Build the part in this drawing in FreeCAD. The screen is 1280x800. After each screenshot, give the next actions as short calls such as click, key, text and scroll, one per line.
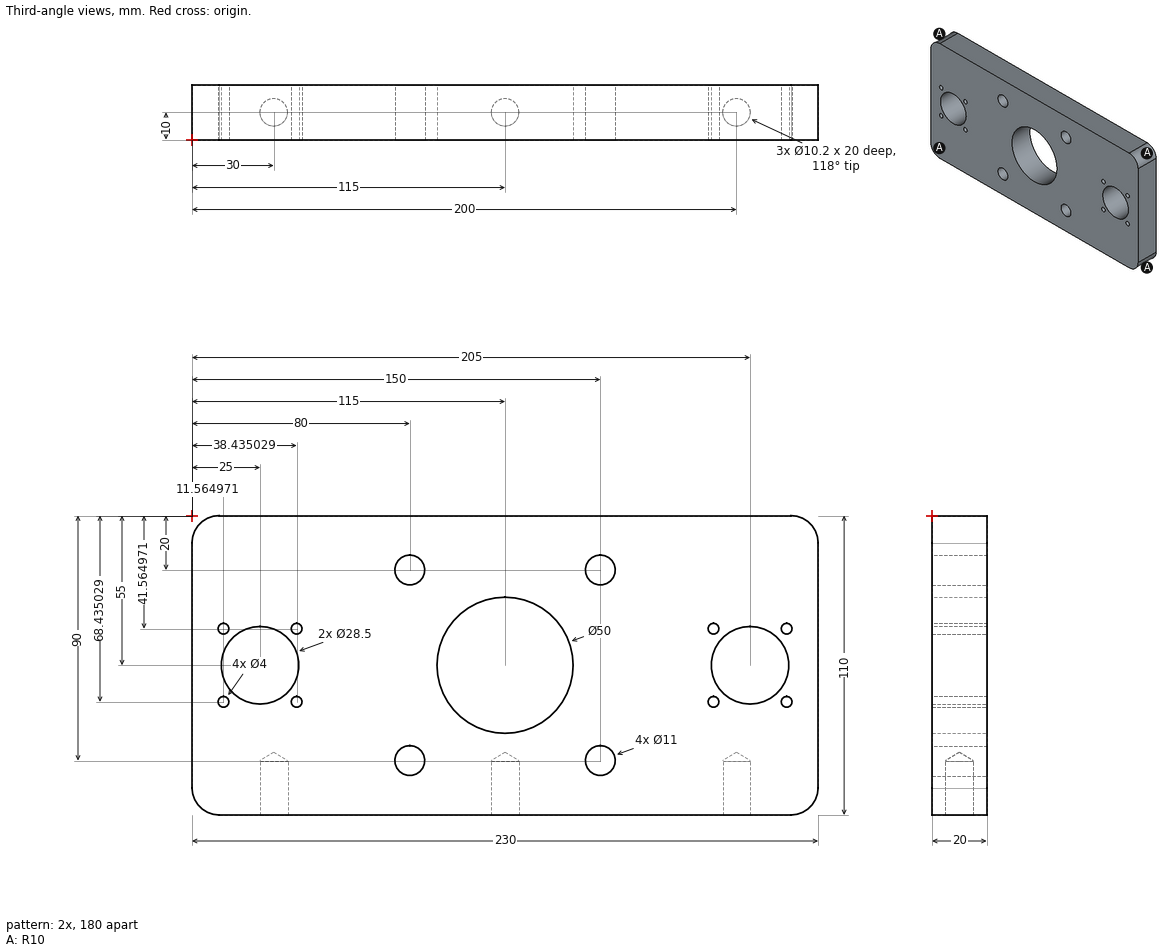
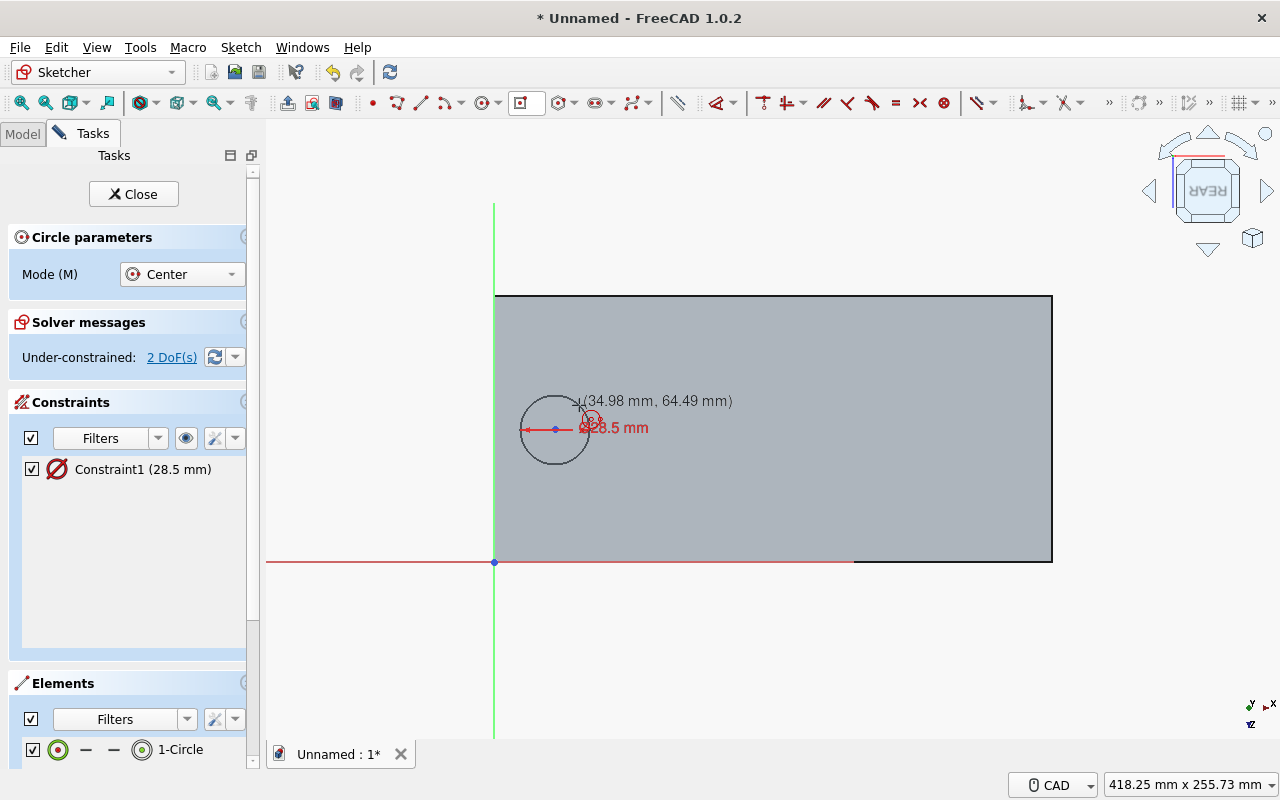
click(991, 429)
move(1016, 405)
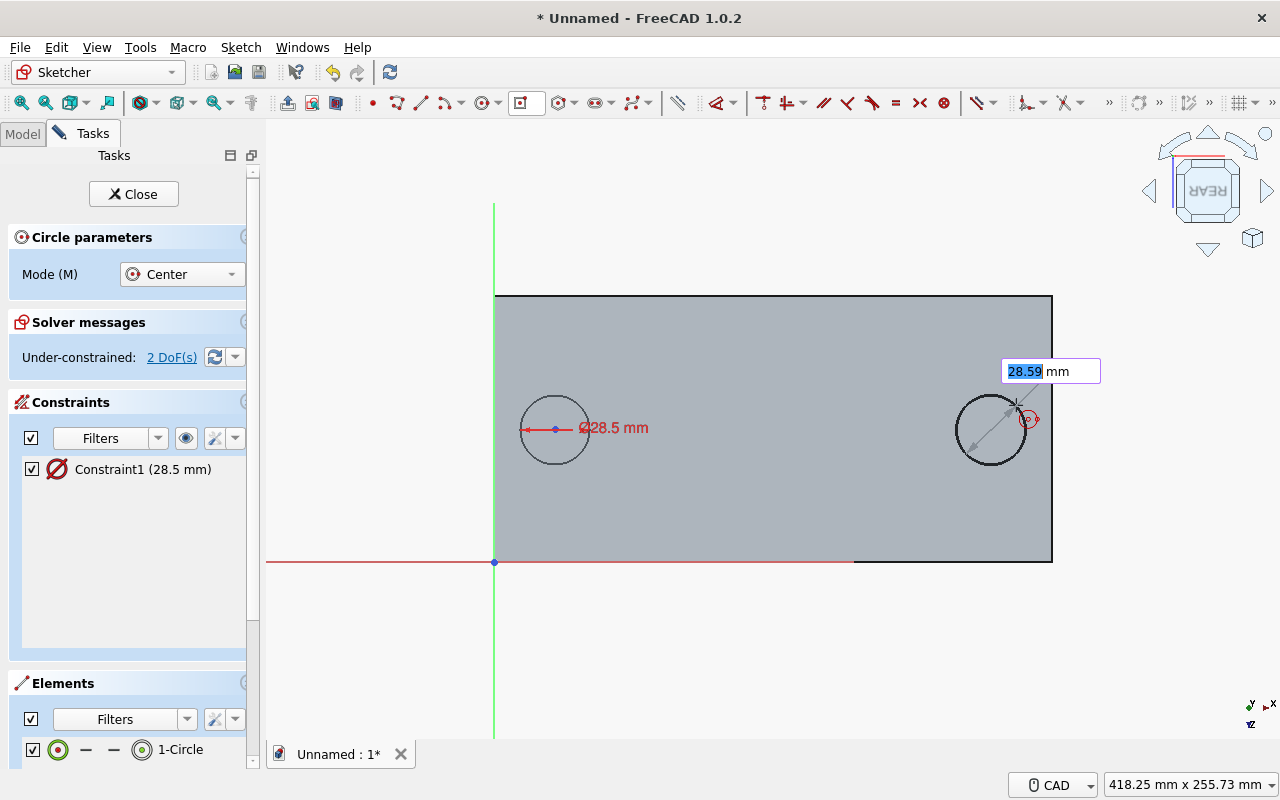
text(28.5)
key(Return)
key(Escape)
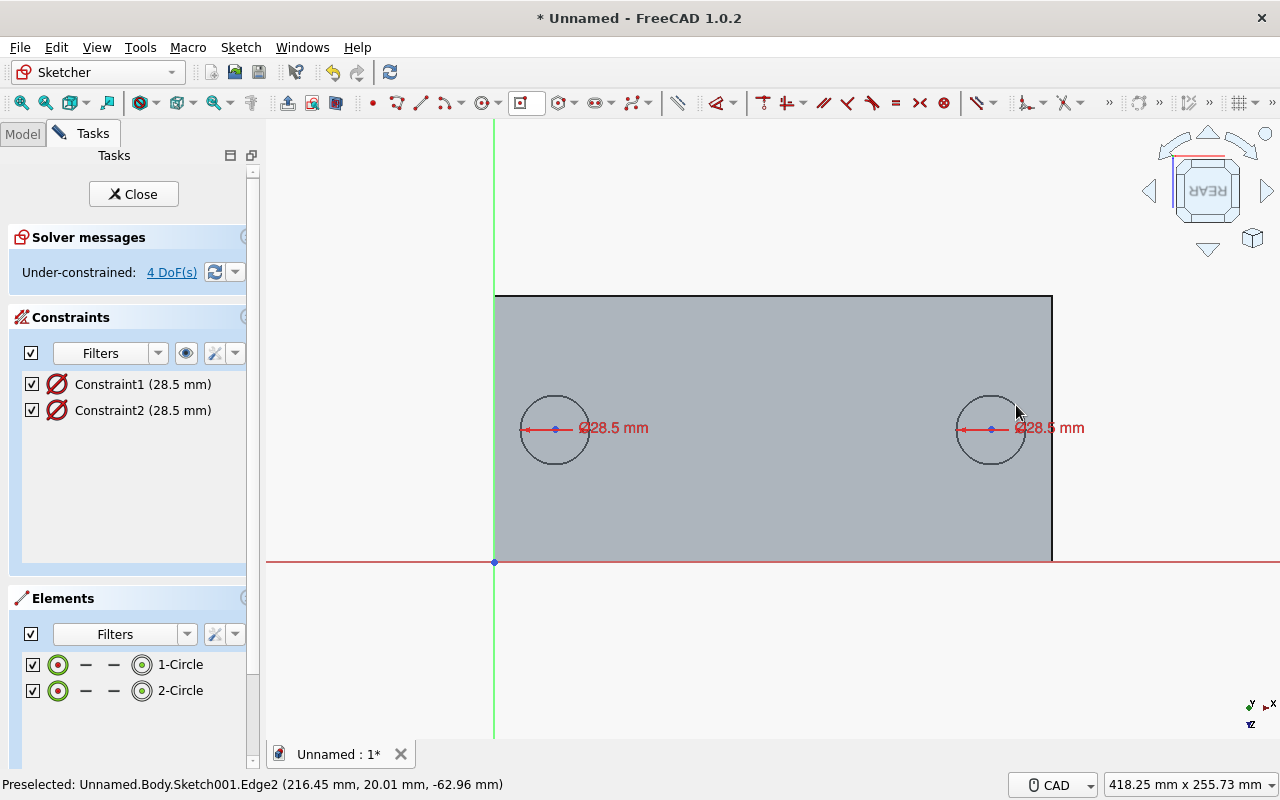
key(d)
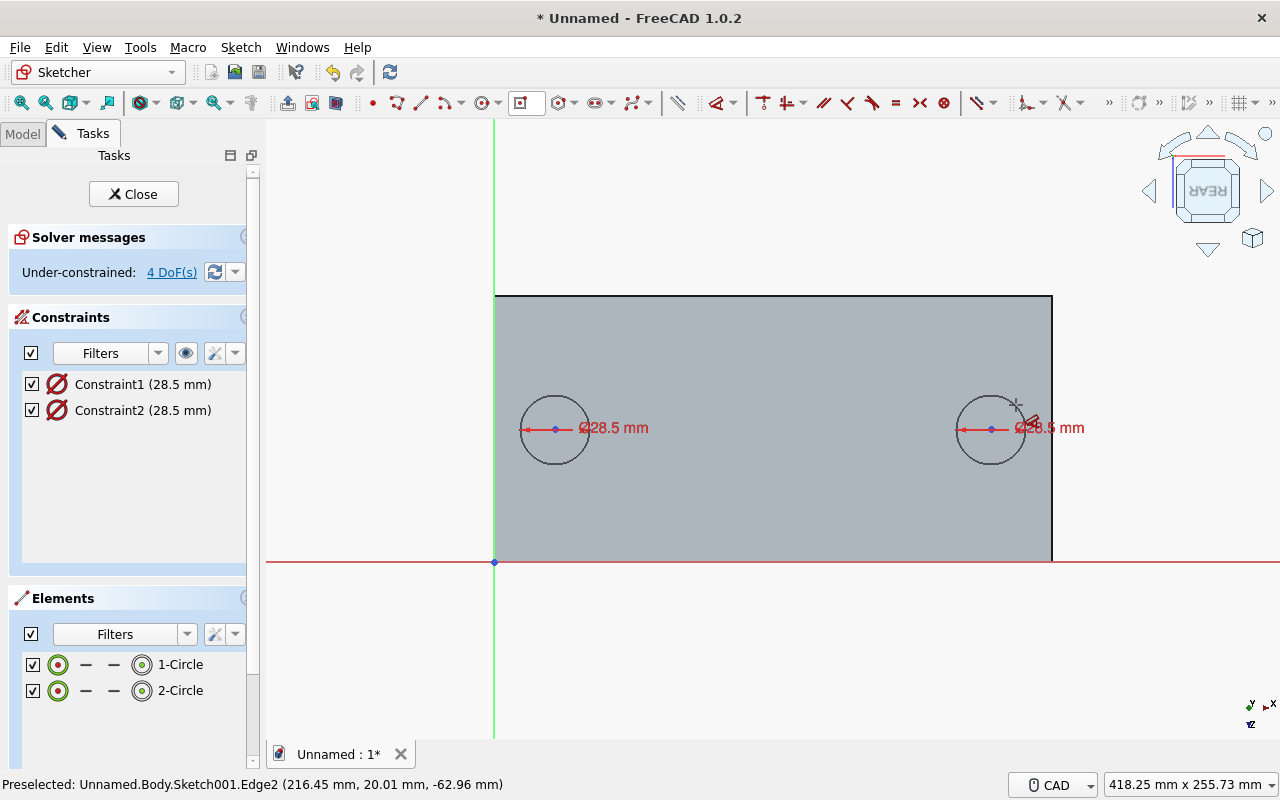
click(555, 430)
click(525, 596)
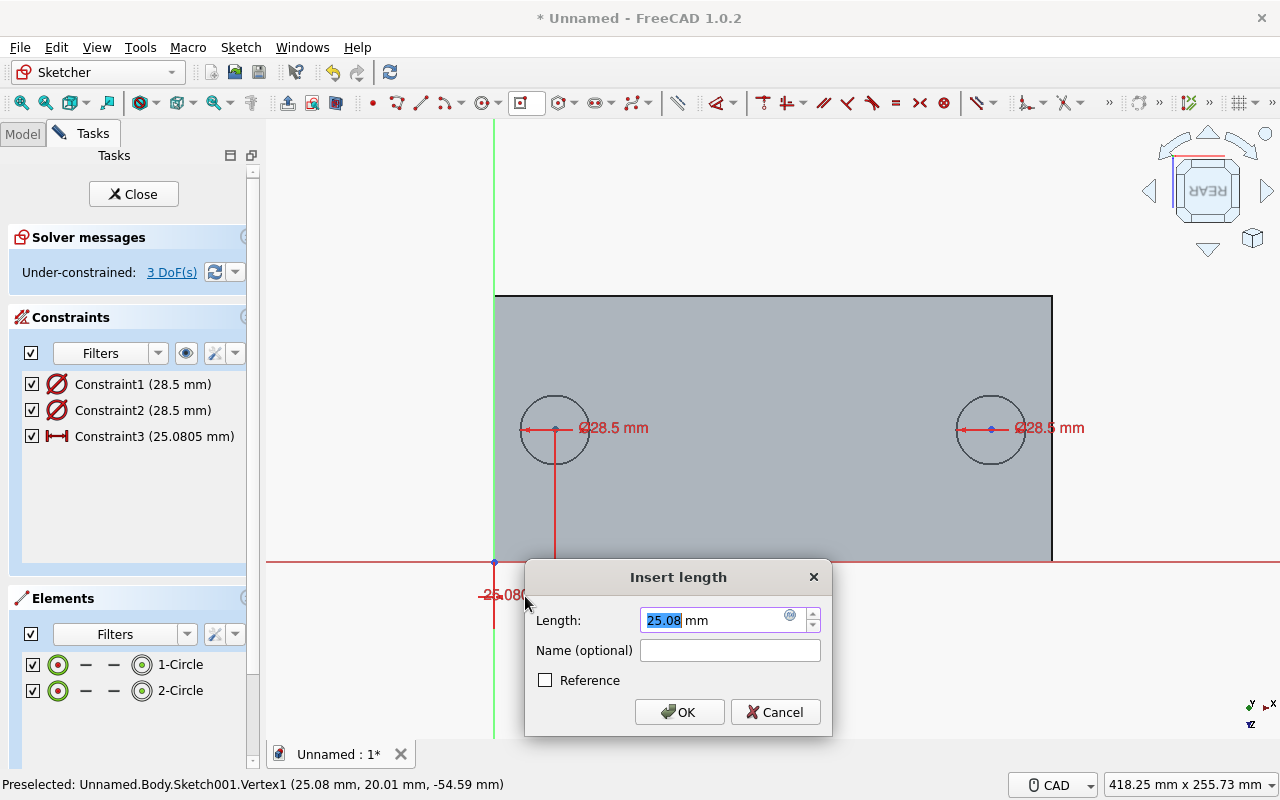
text(25)
key(Return)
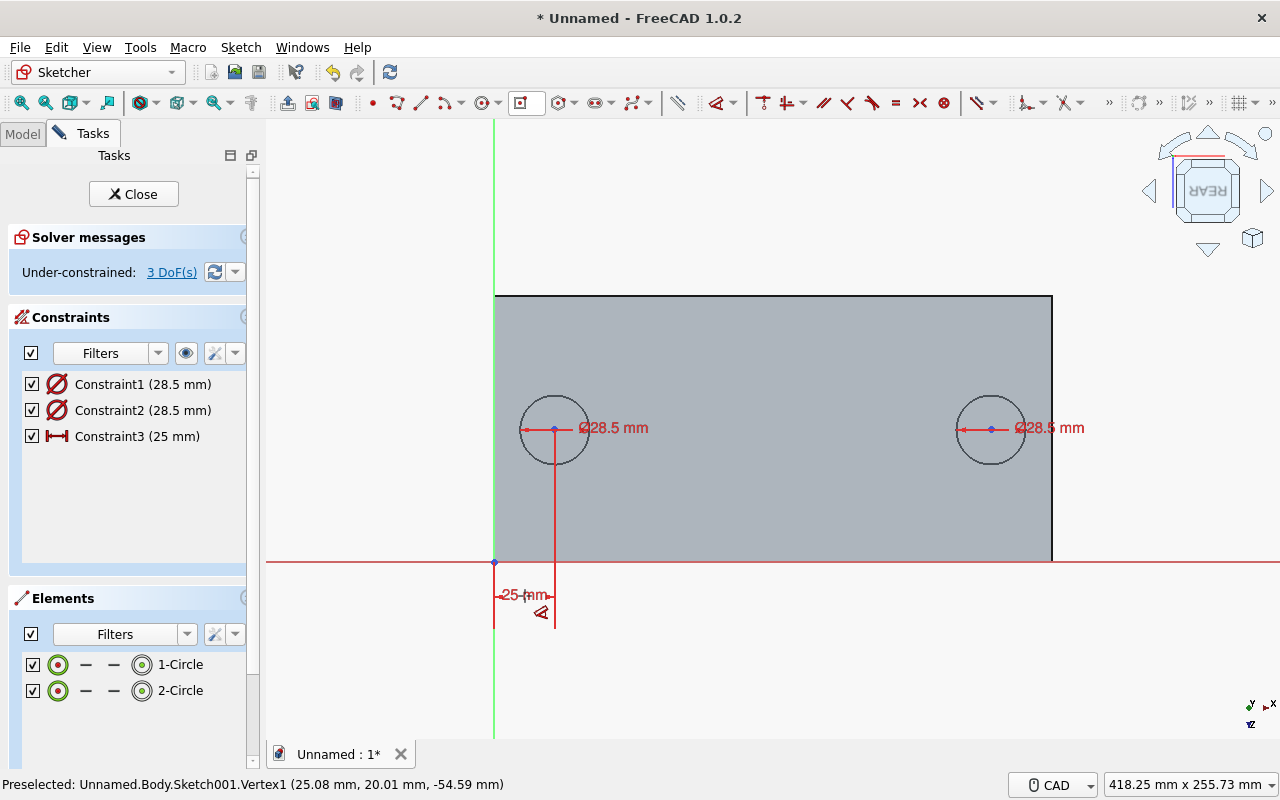
click(555, 430)
click(460, 496)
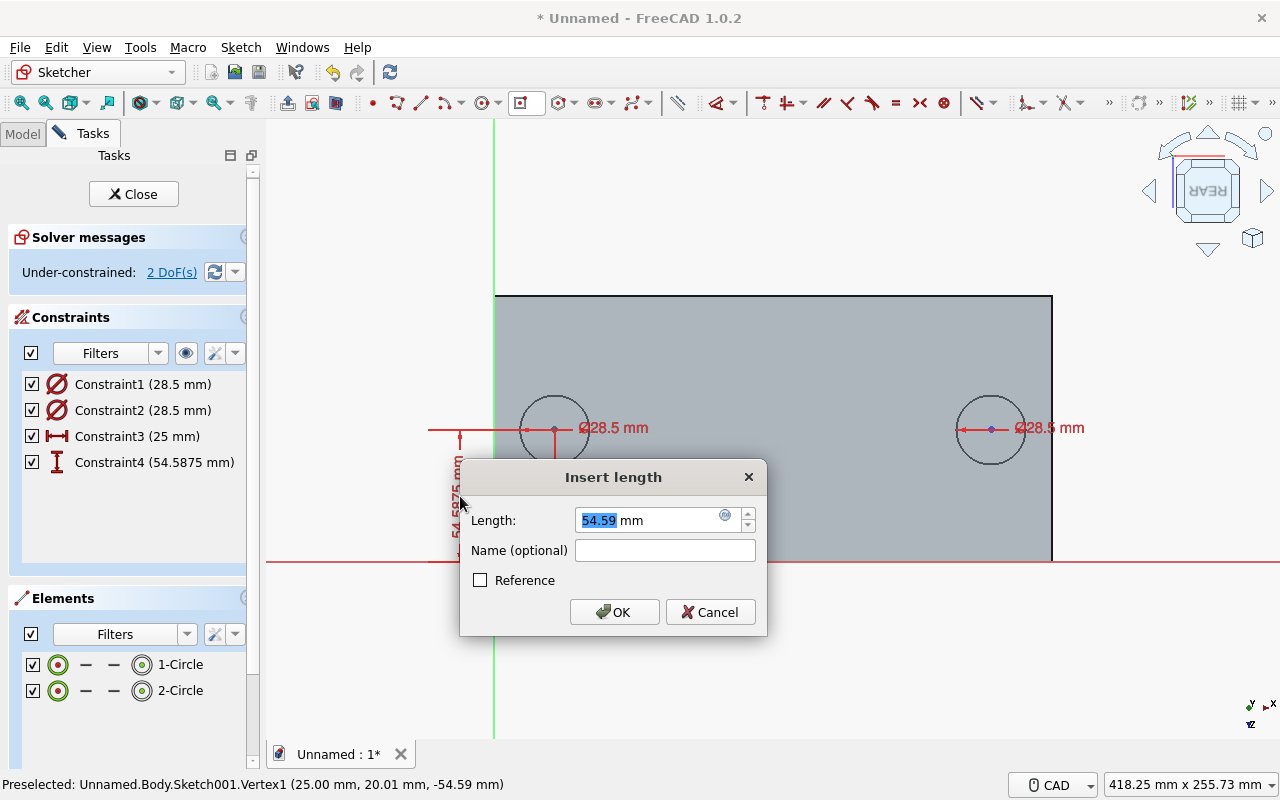
text(55)
key(Return)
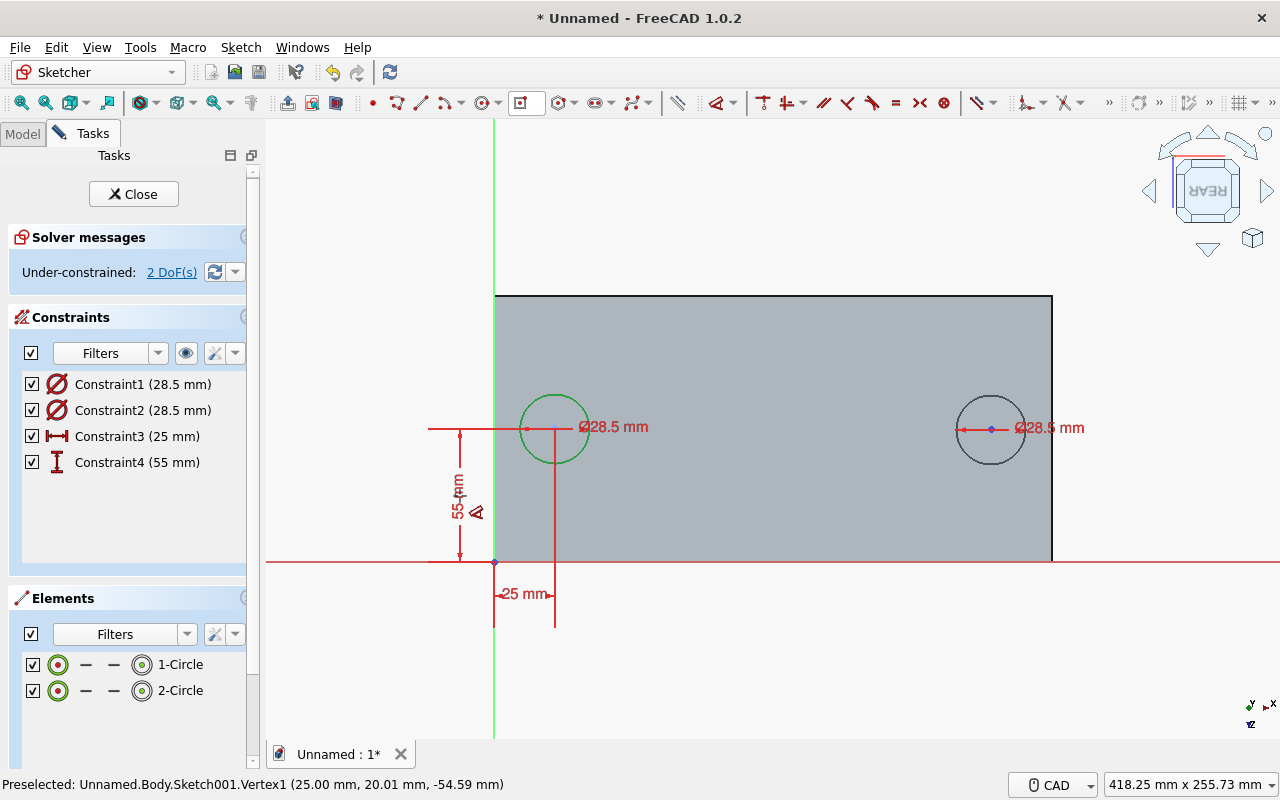
click(991, 430)
click(460, 466)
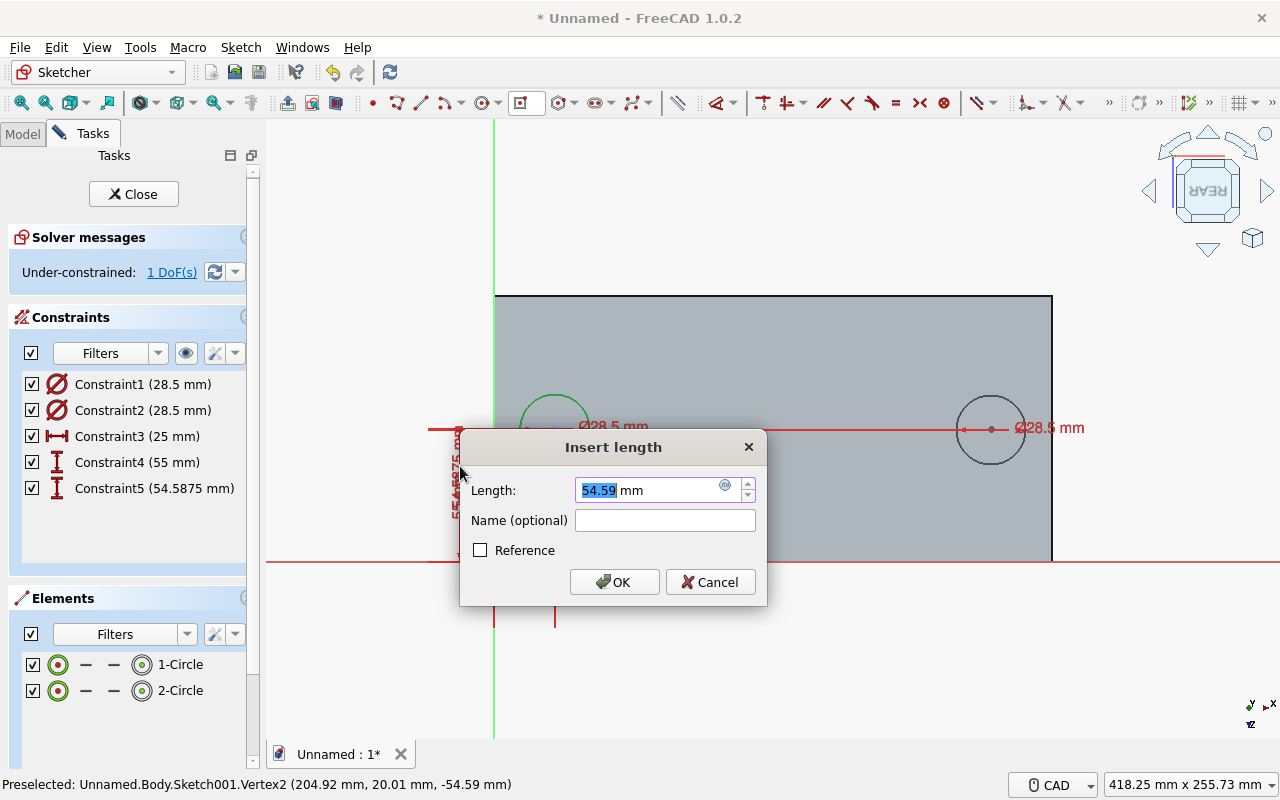
text(55)
key(Return)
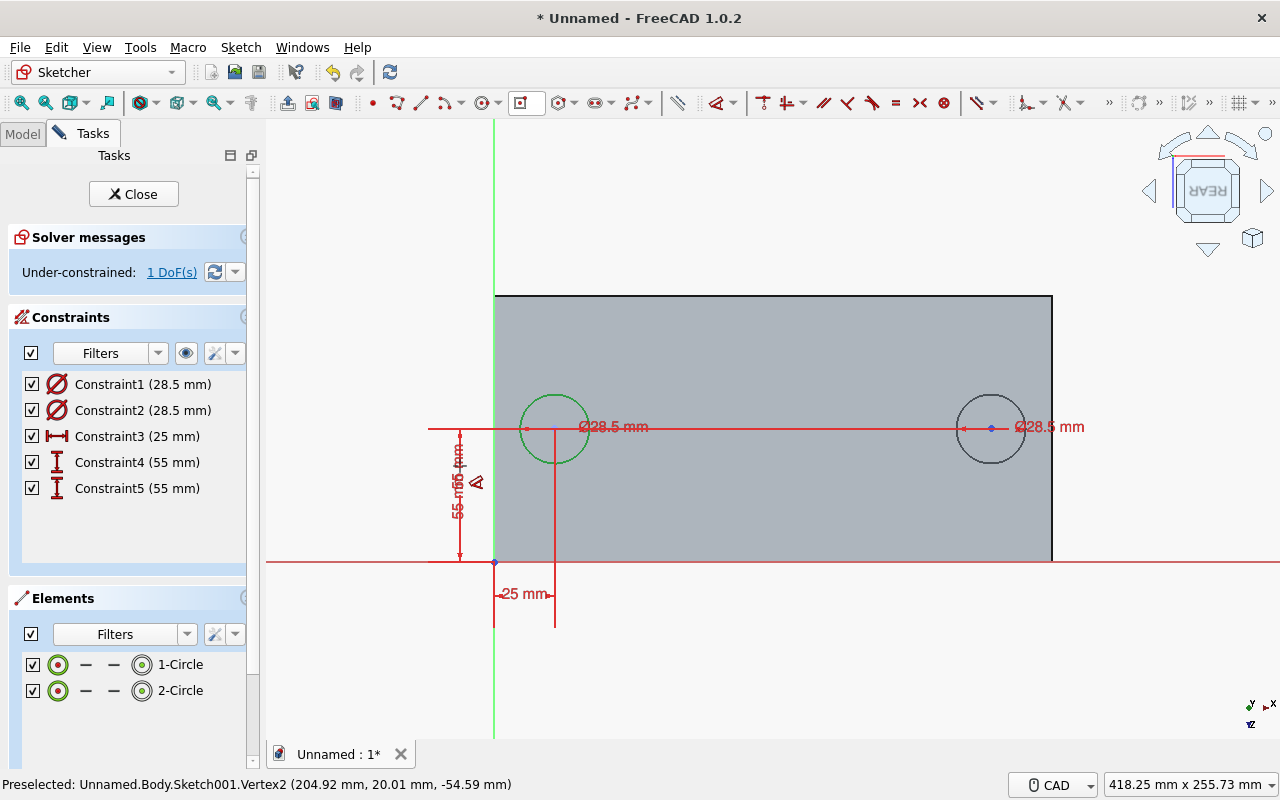
click(991, 429)
click(743, 596)